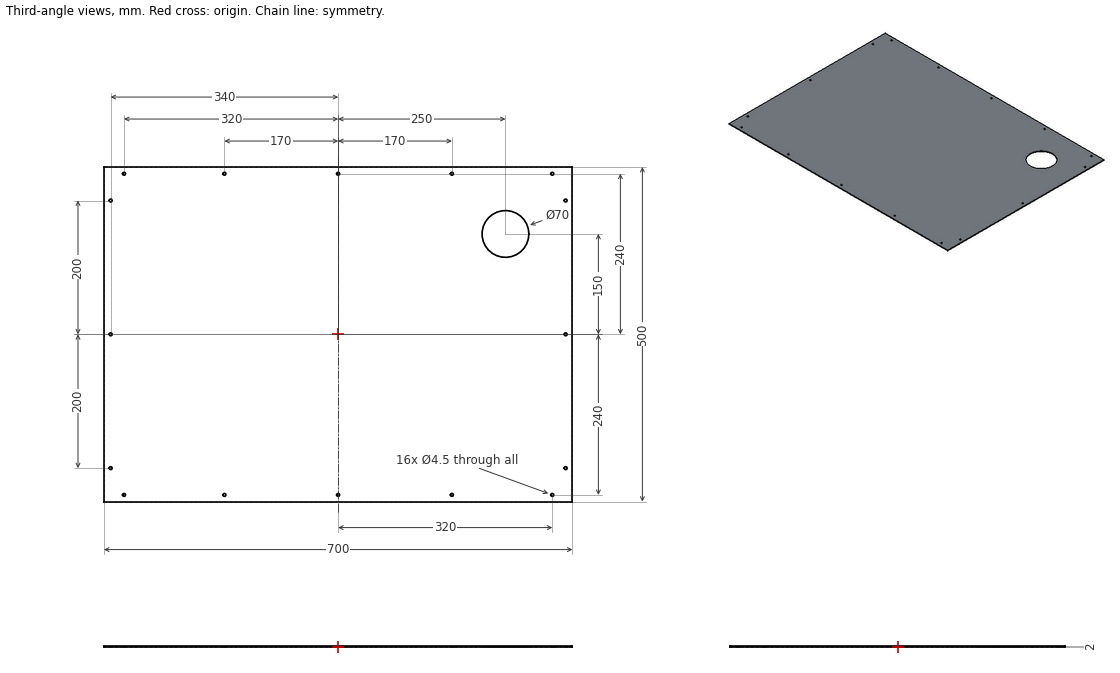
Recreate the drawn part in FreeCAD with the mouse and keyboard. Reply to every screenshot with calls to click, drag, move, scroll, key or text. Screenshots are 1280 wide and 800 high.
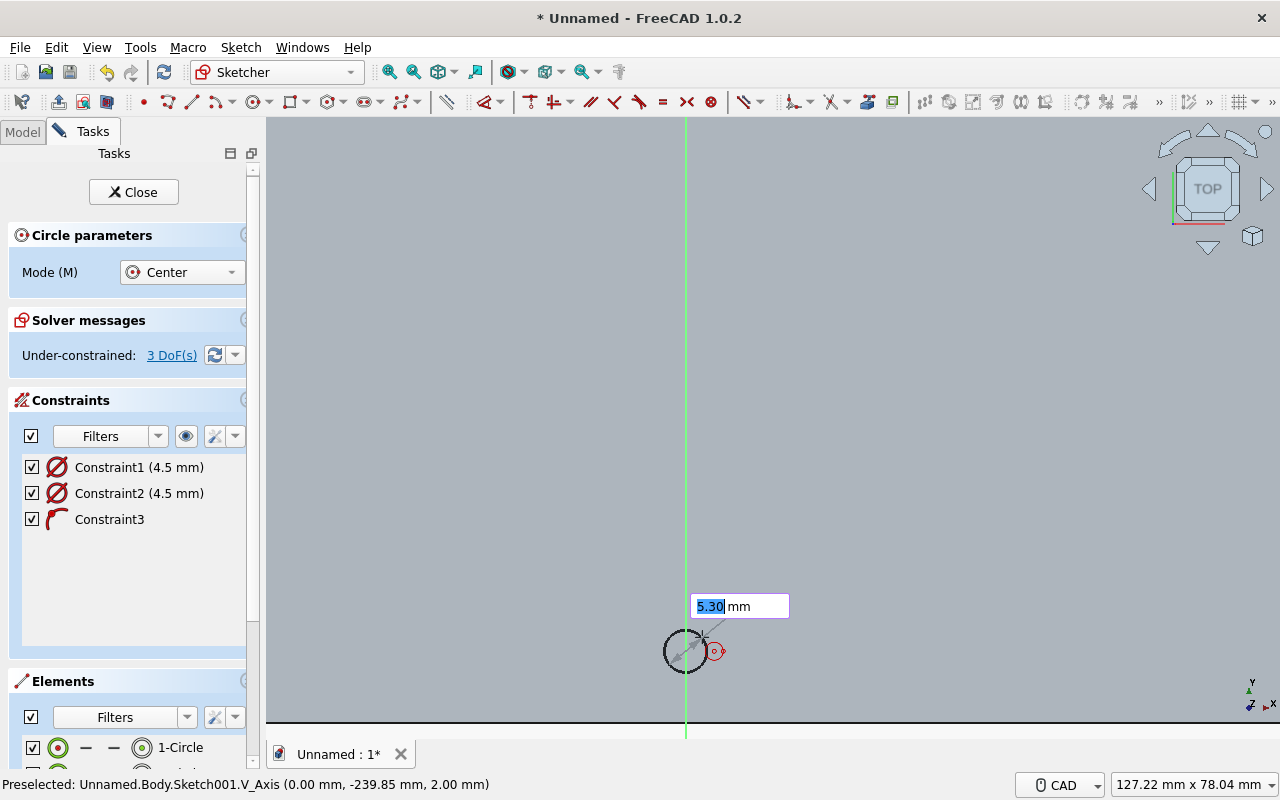
text(4.5)
key(Return)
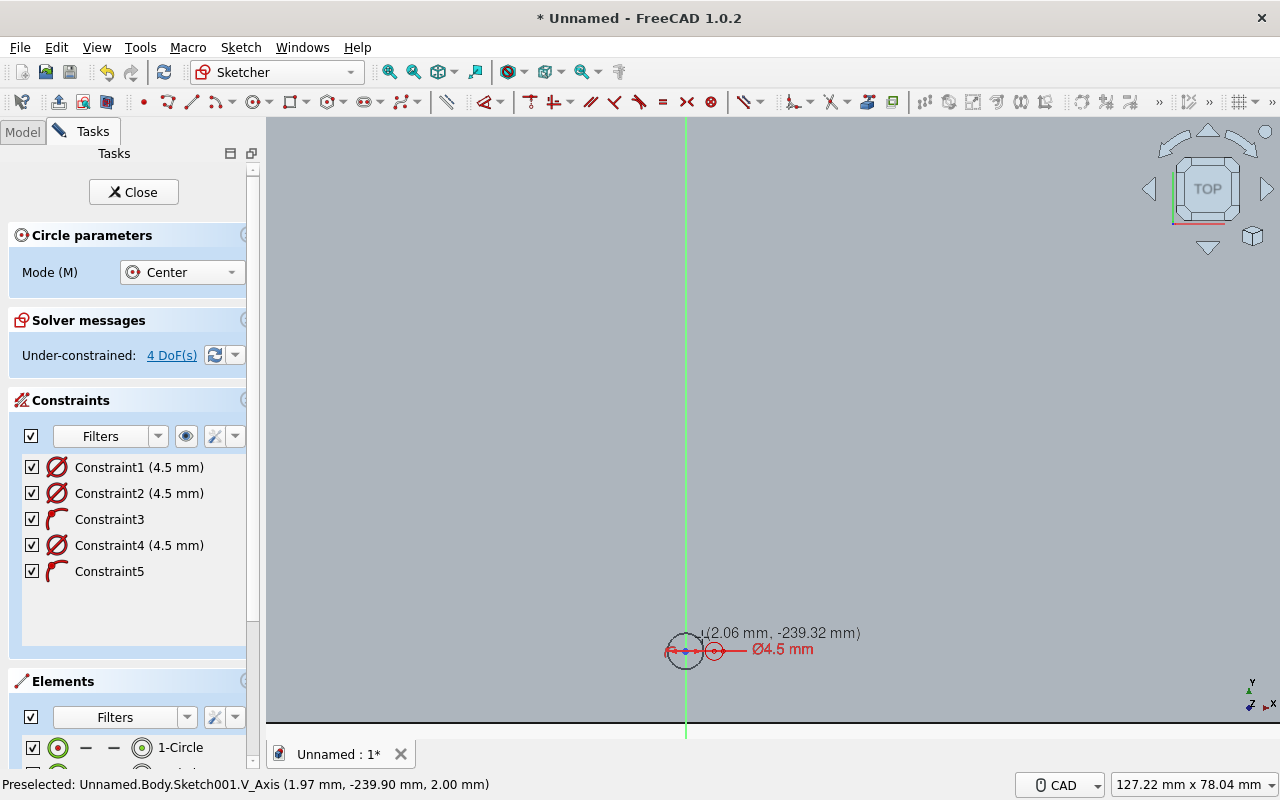
scroll(707, 640, down, 11)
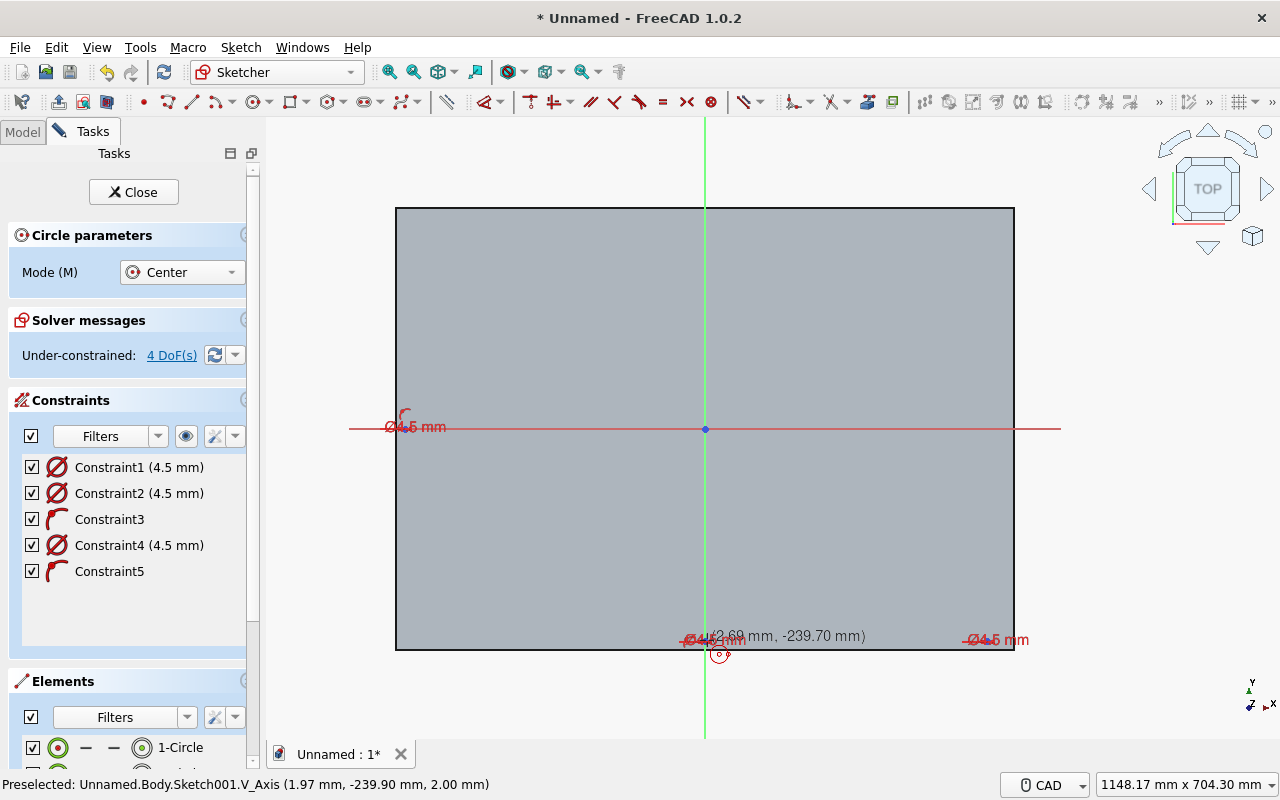
scroll(1005, 429, up, 13)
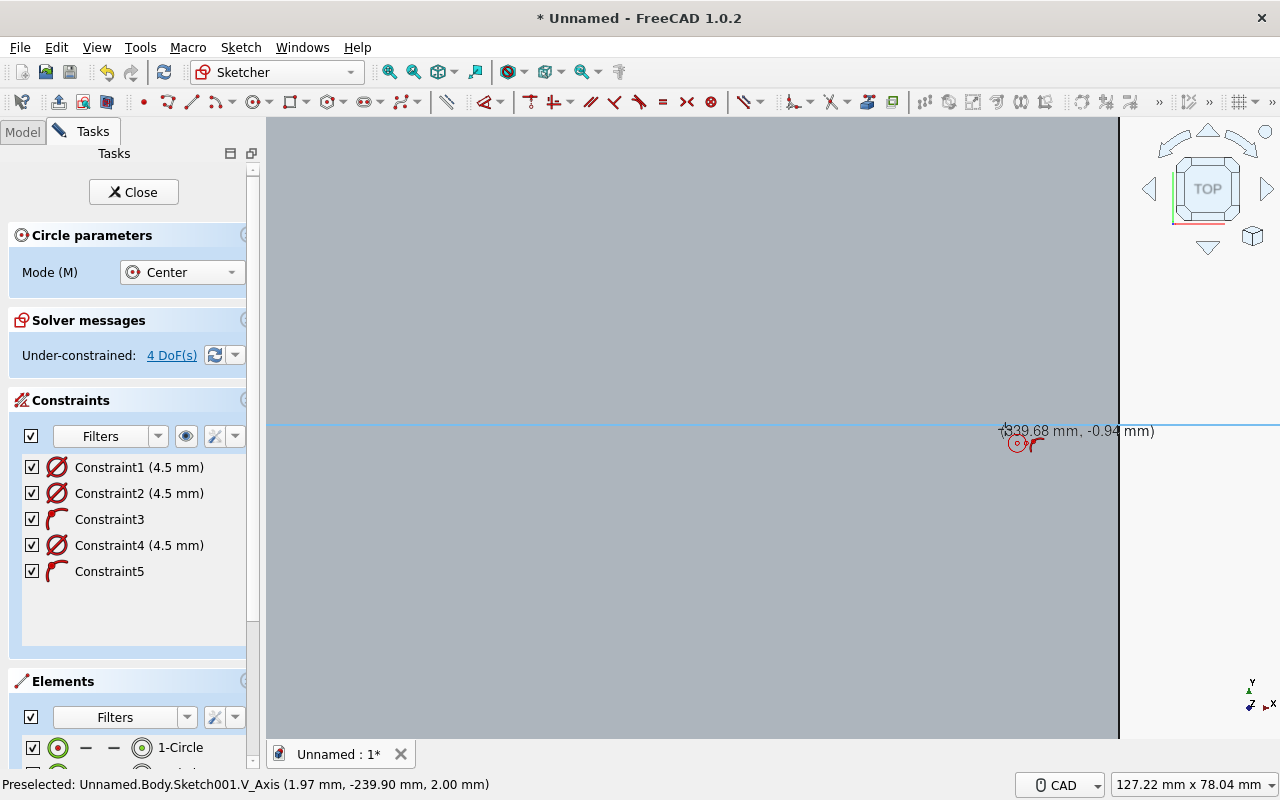
scroll(1005, 428, down, 13)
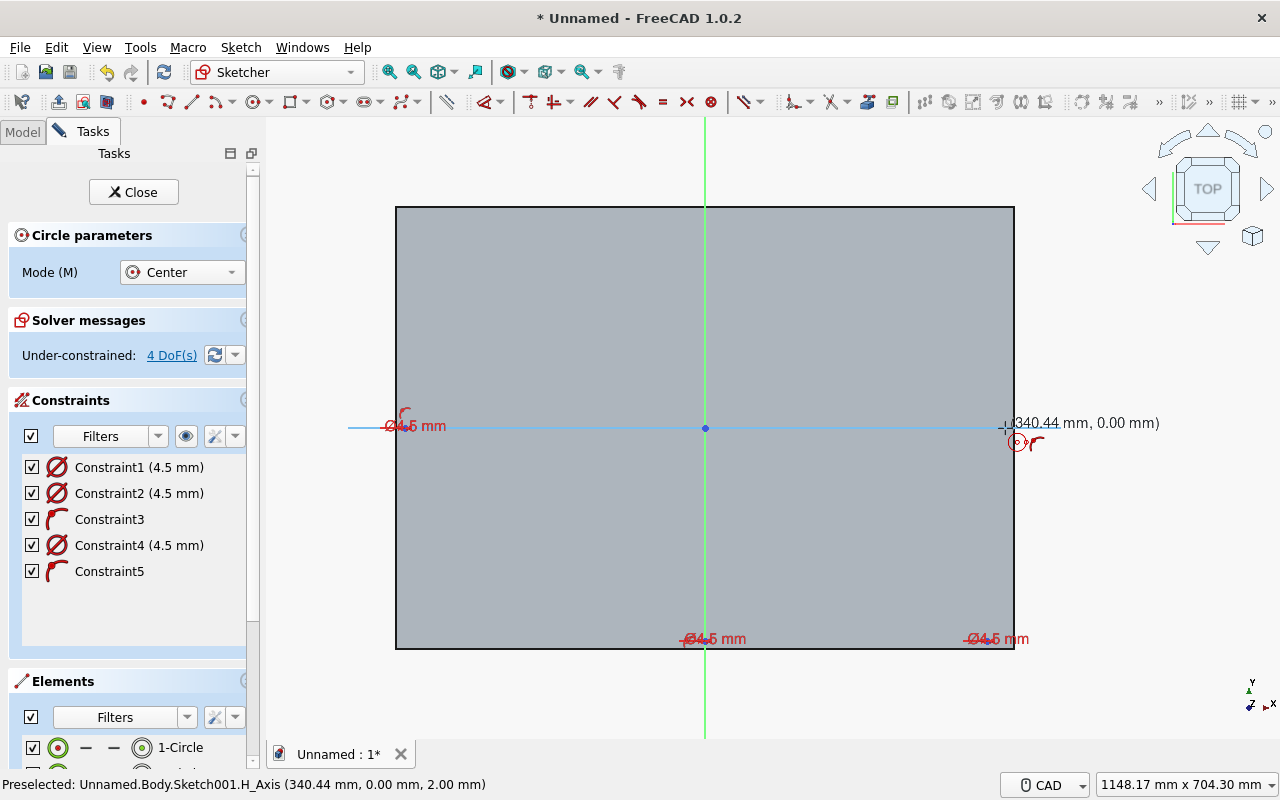
click(1005, 428)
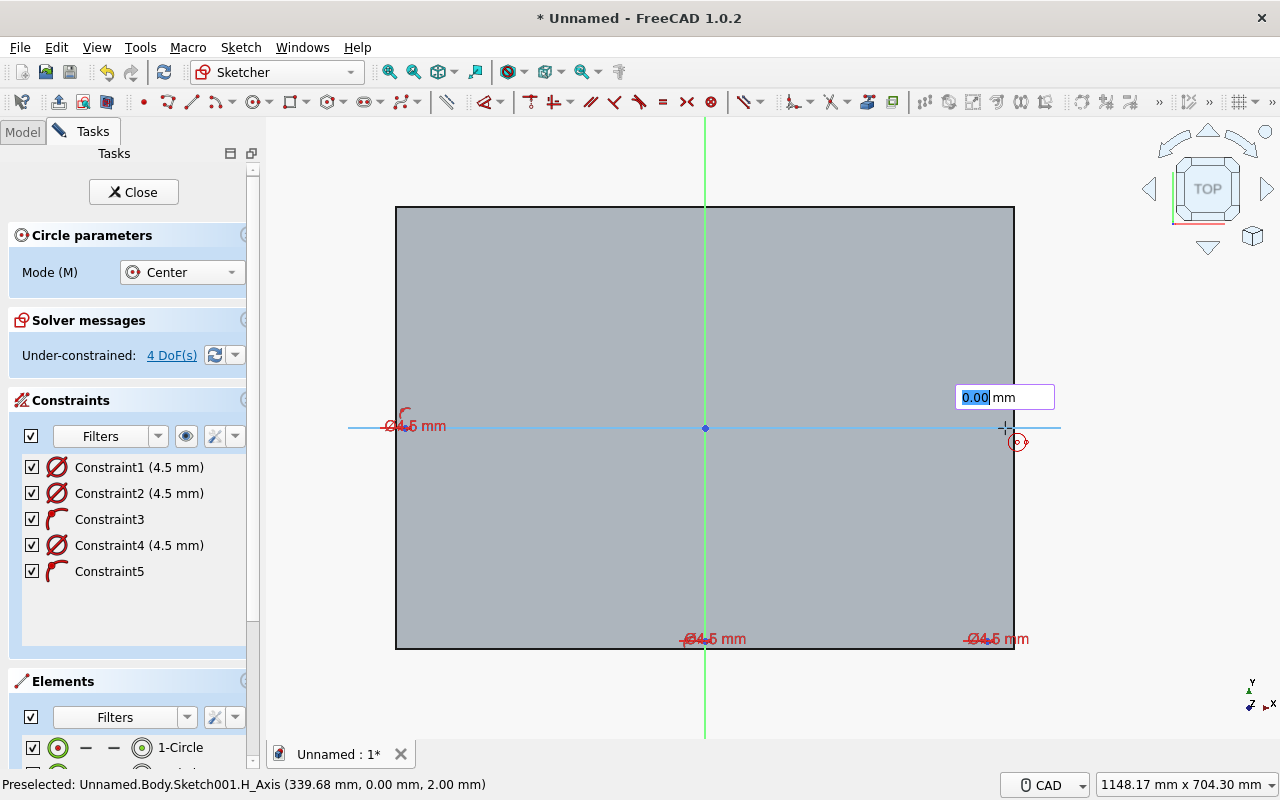
scroll(1005, 430, up, 11)
move(996, 427)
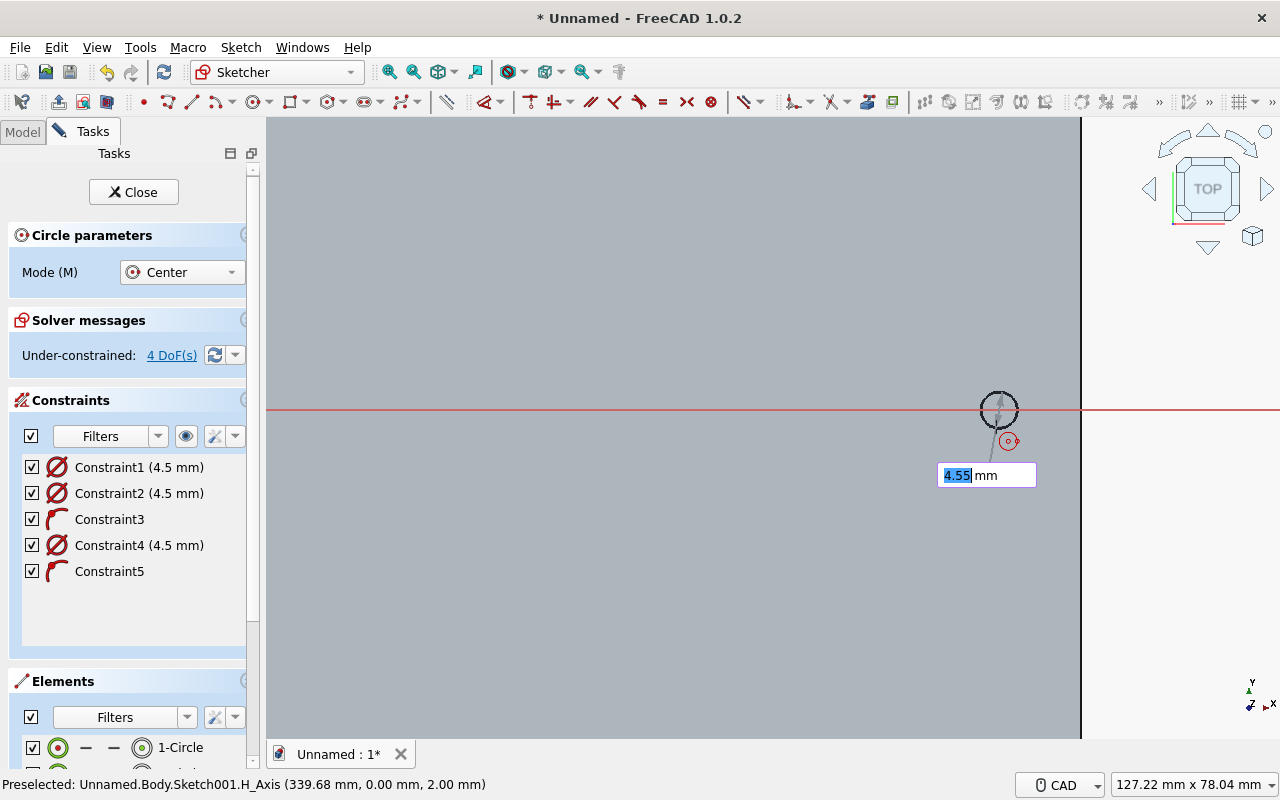
text(4.5)
key(Return)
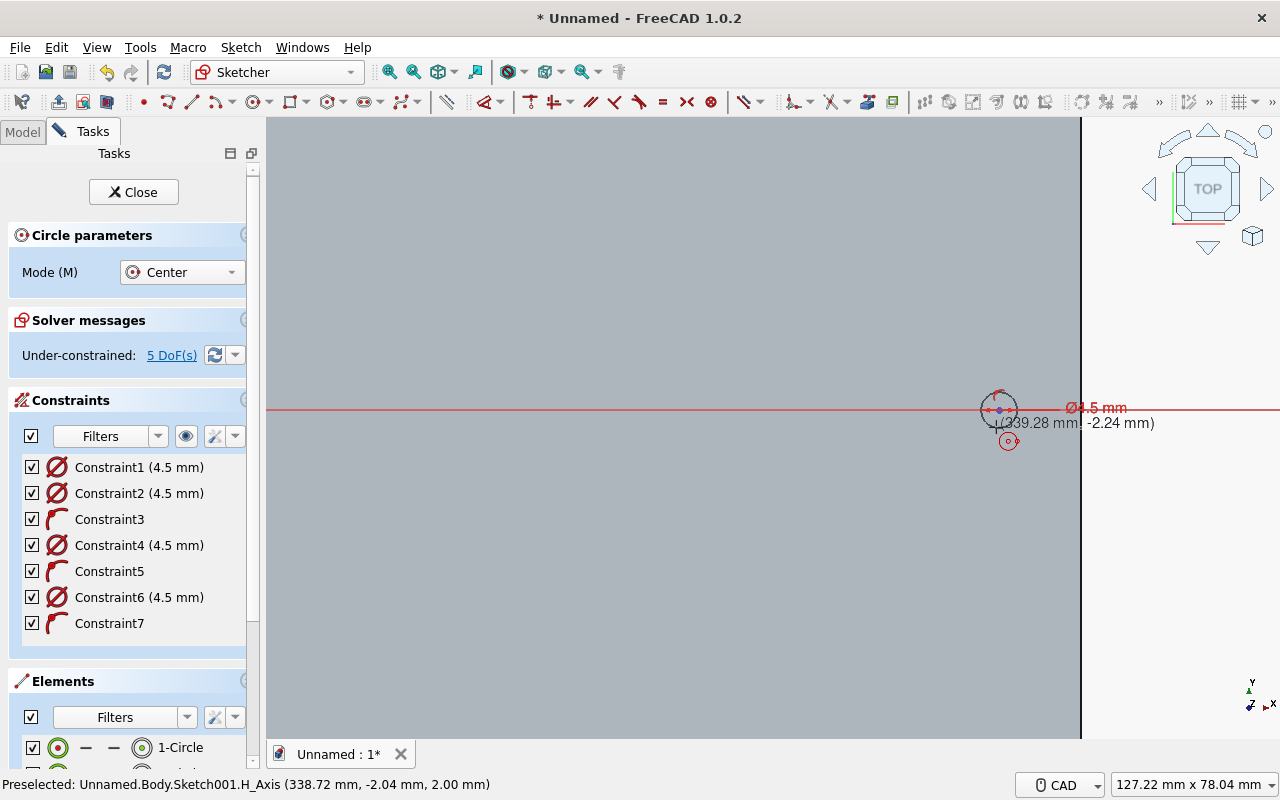
scroll(1005, 430, down, 11)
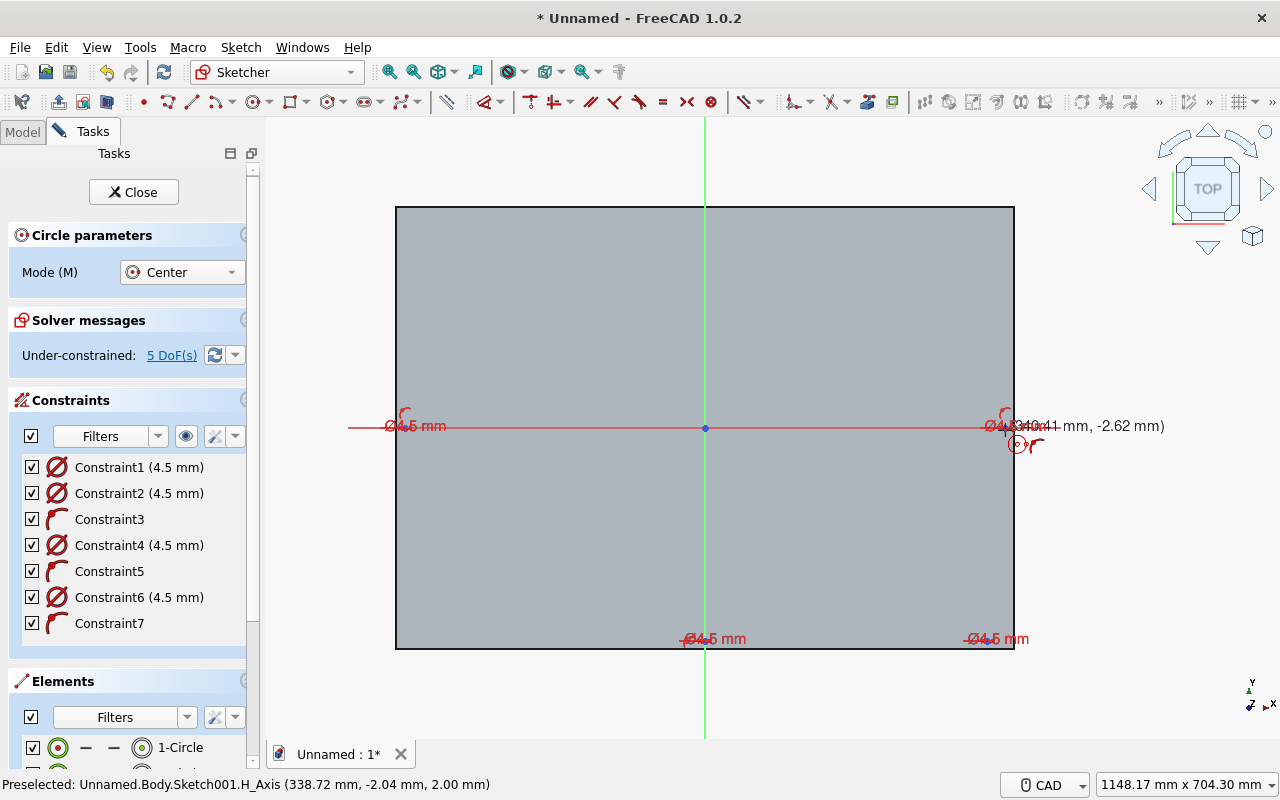
scroll(705, 216, up, 13)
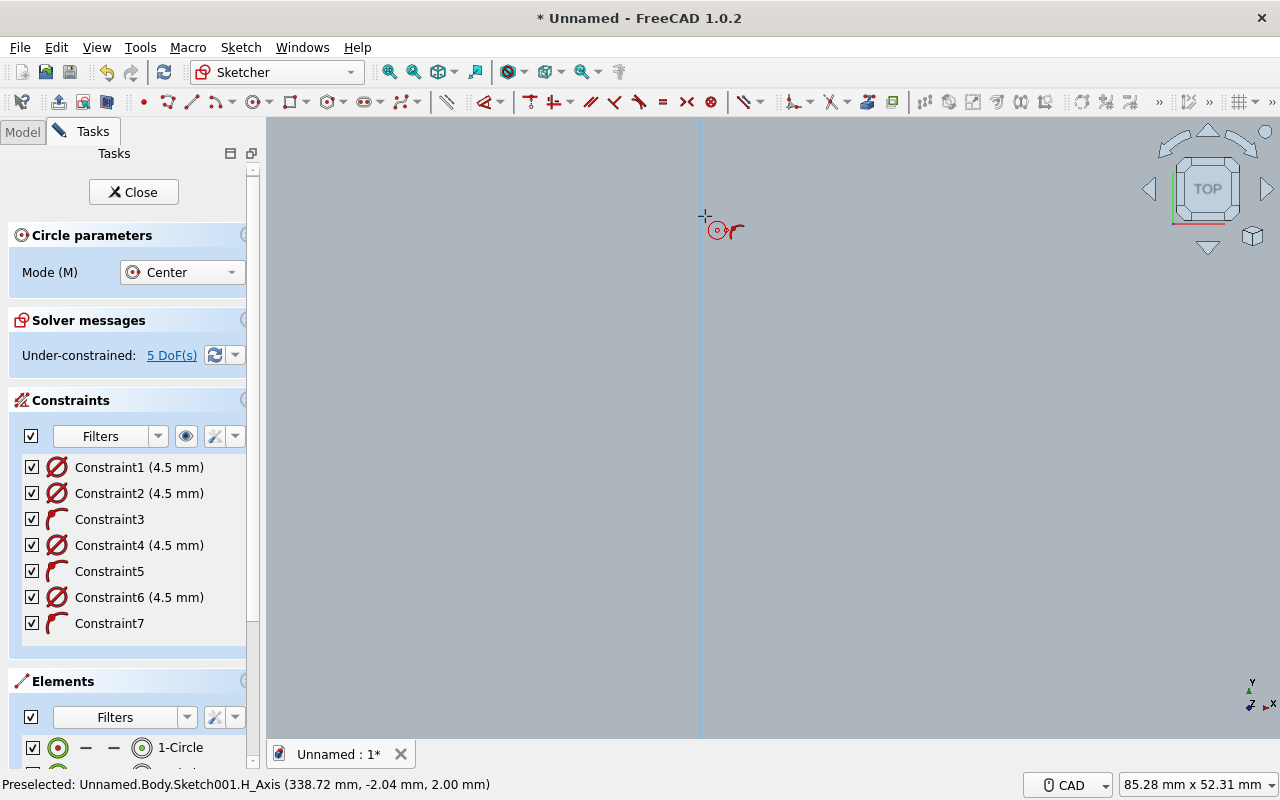
scroll(705, 216, down, 13)